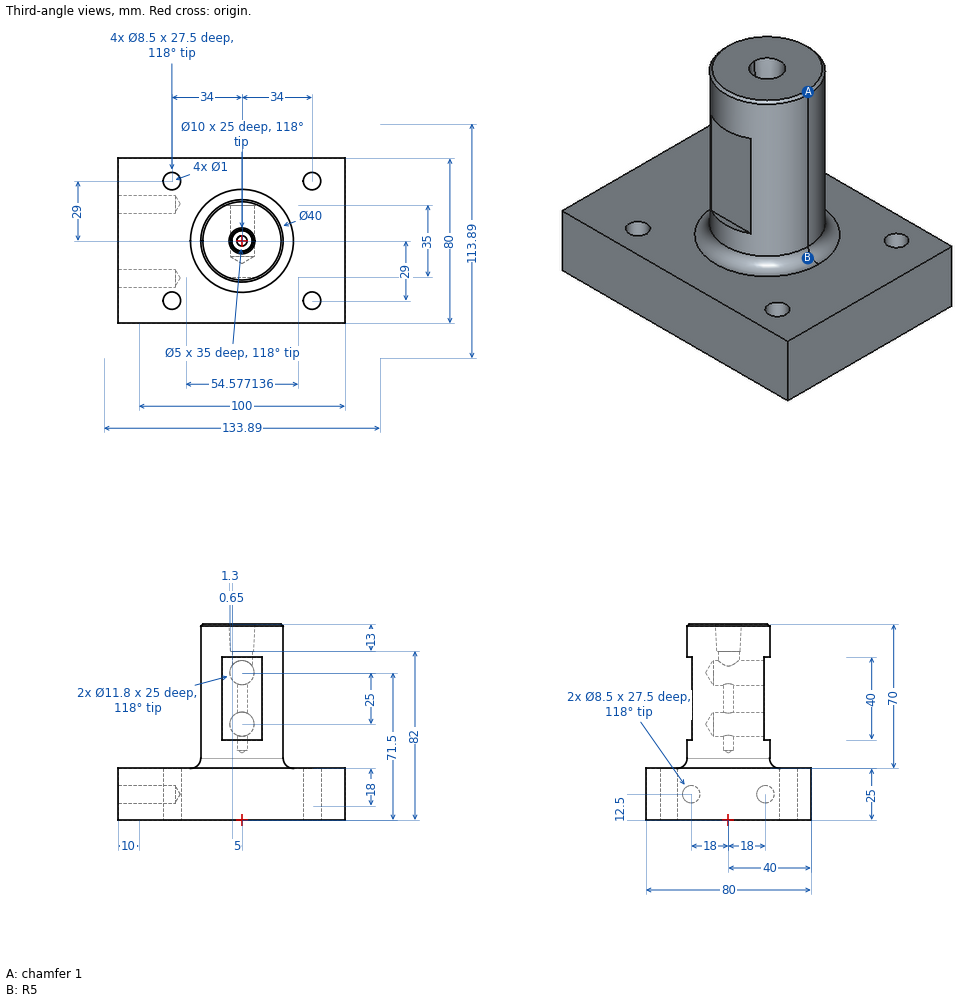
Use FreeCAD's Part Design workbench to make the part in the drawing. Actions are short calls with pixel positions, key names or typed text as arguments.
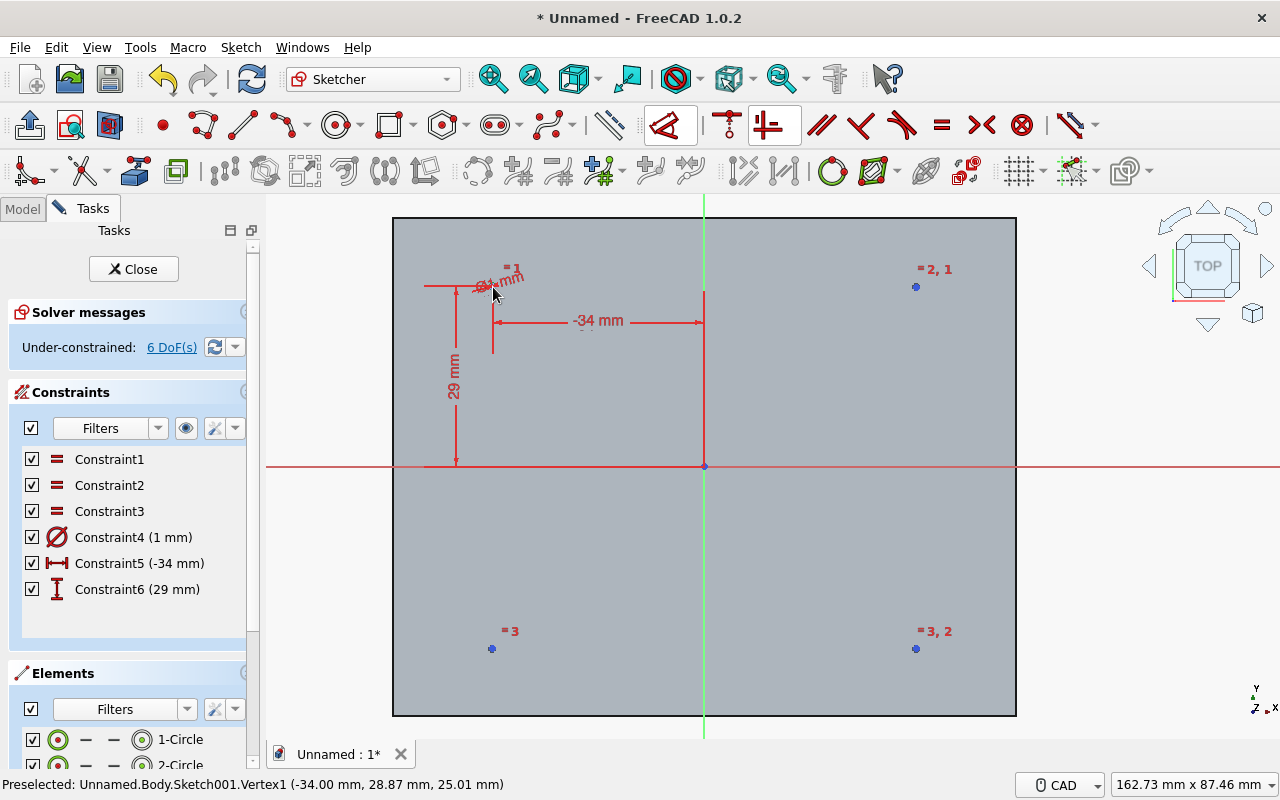
click(916, 287)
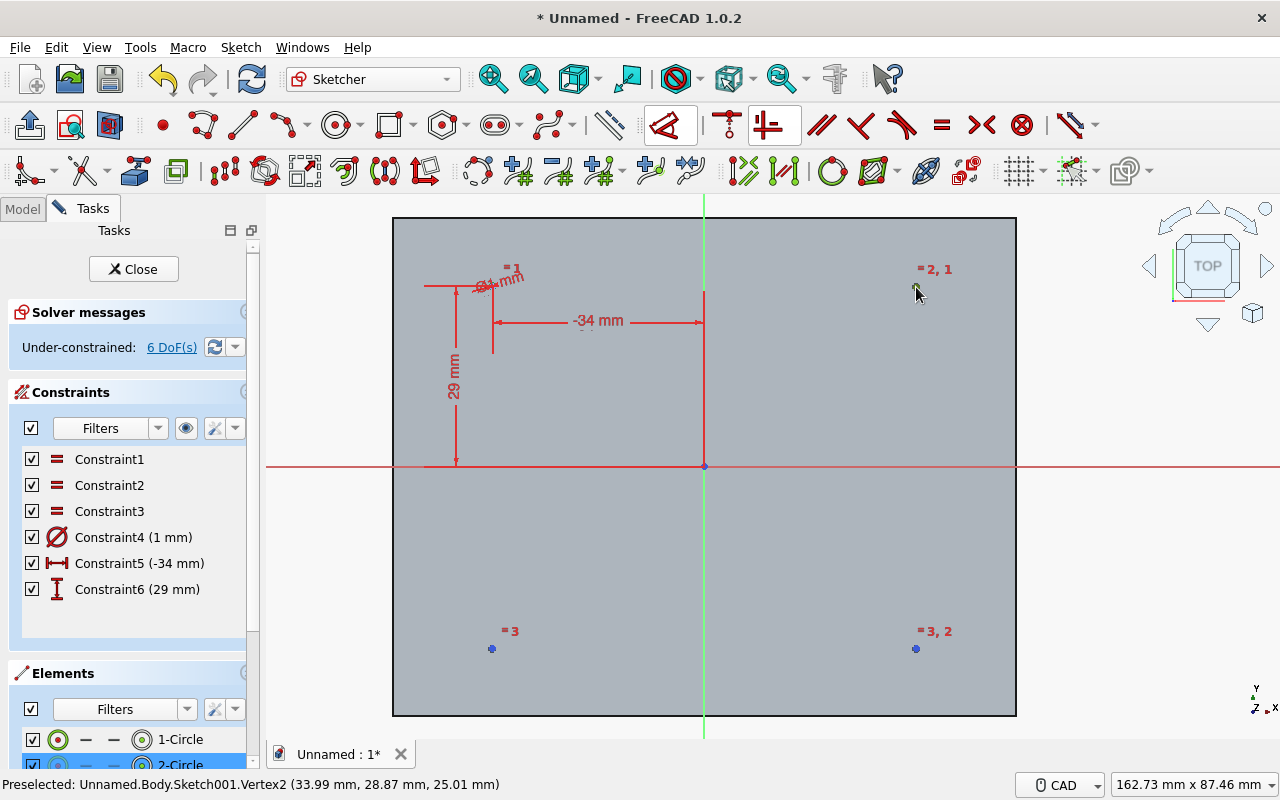
key(l)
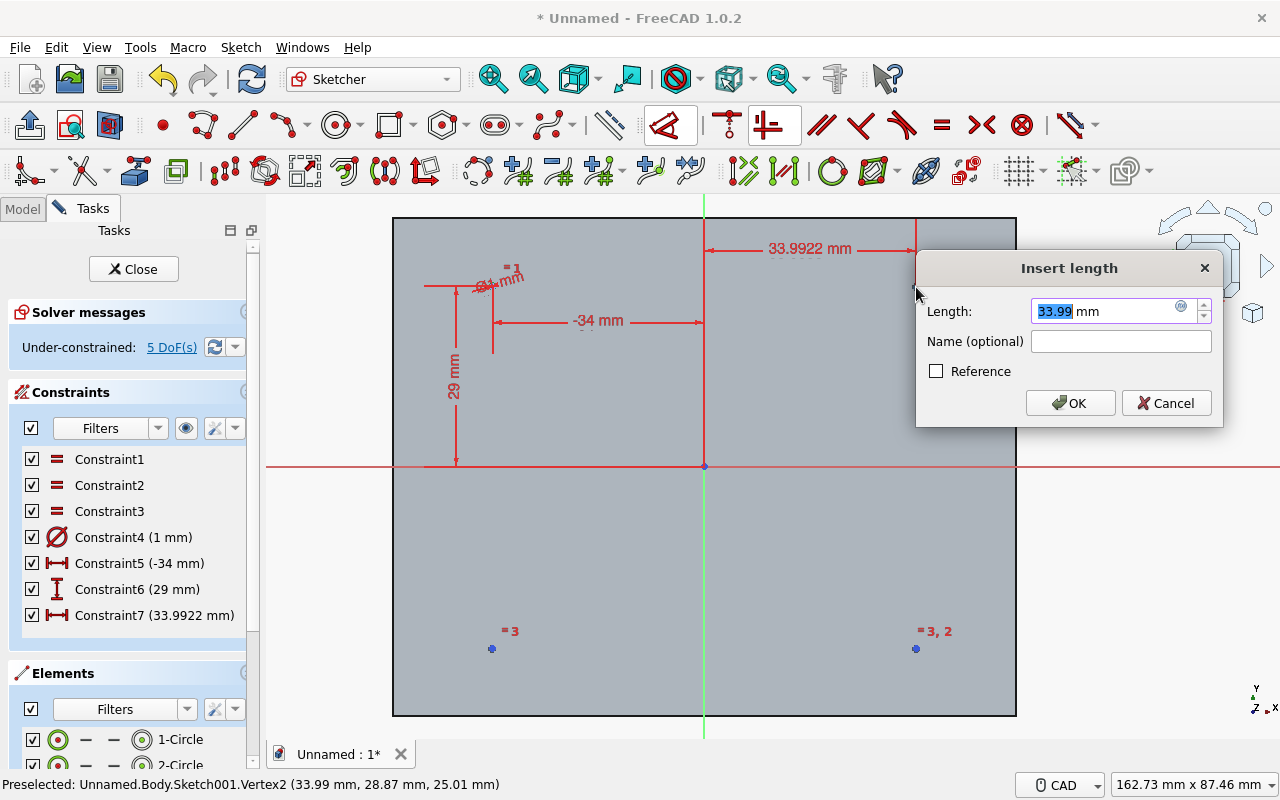
text(34)
key(Return)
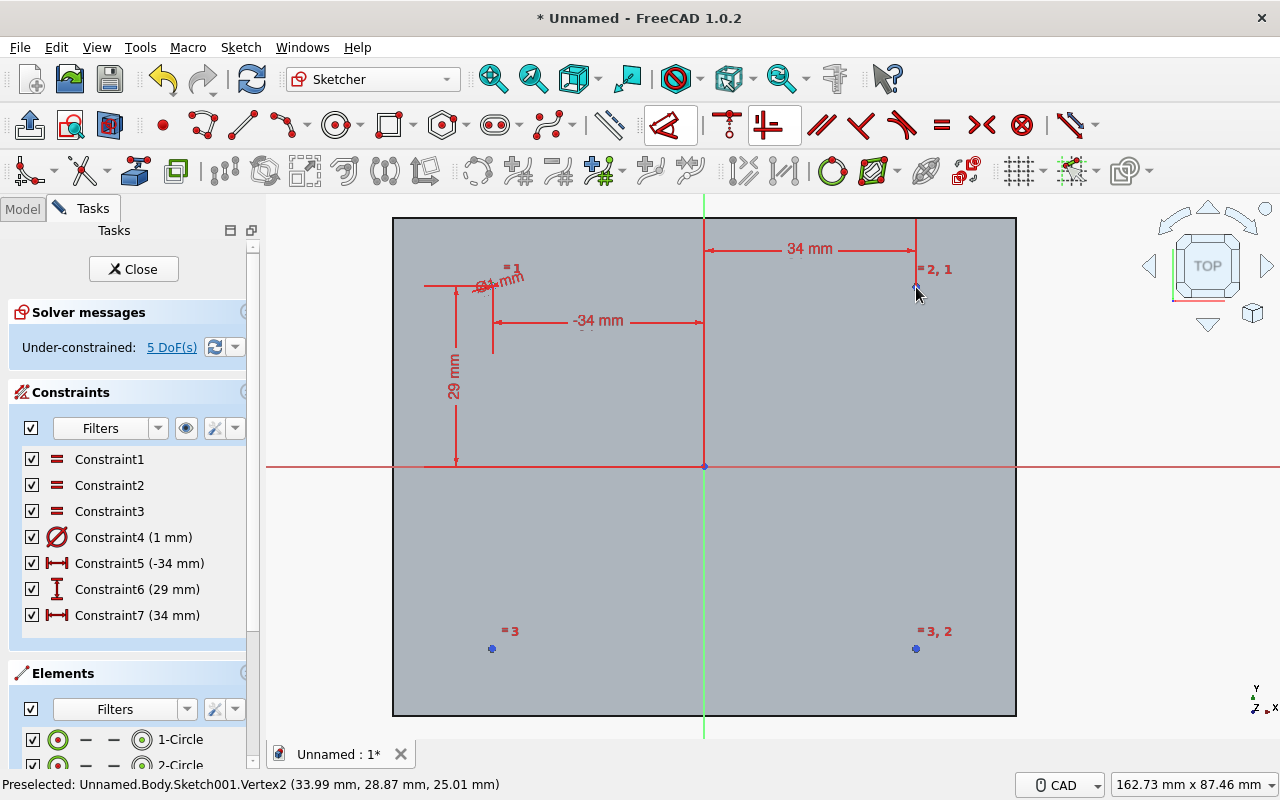
click(916, 287)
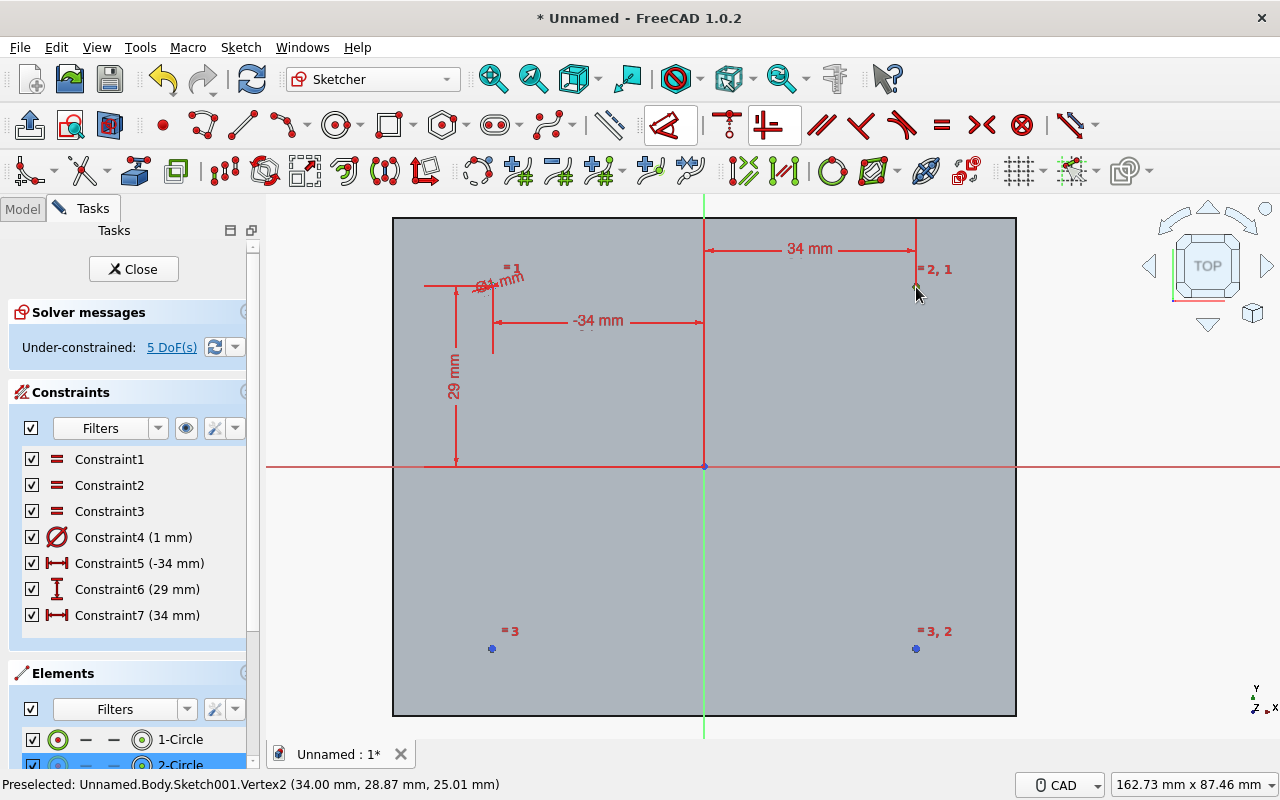
click(692, 126)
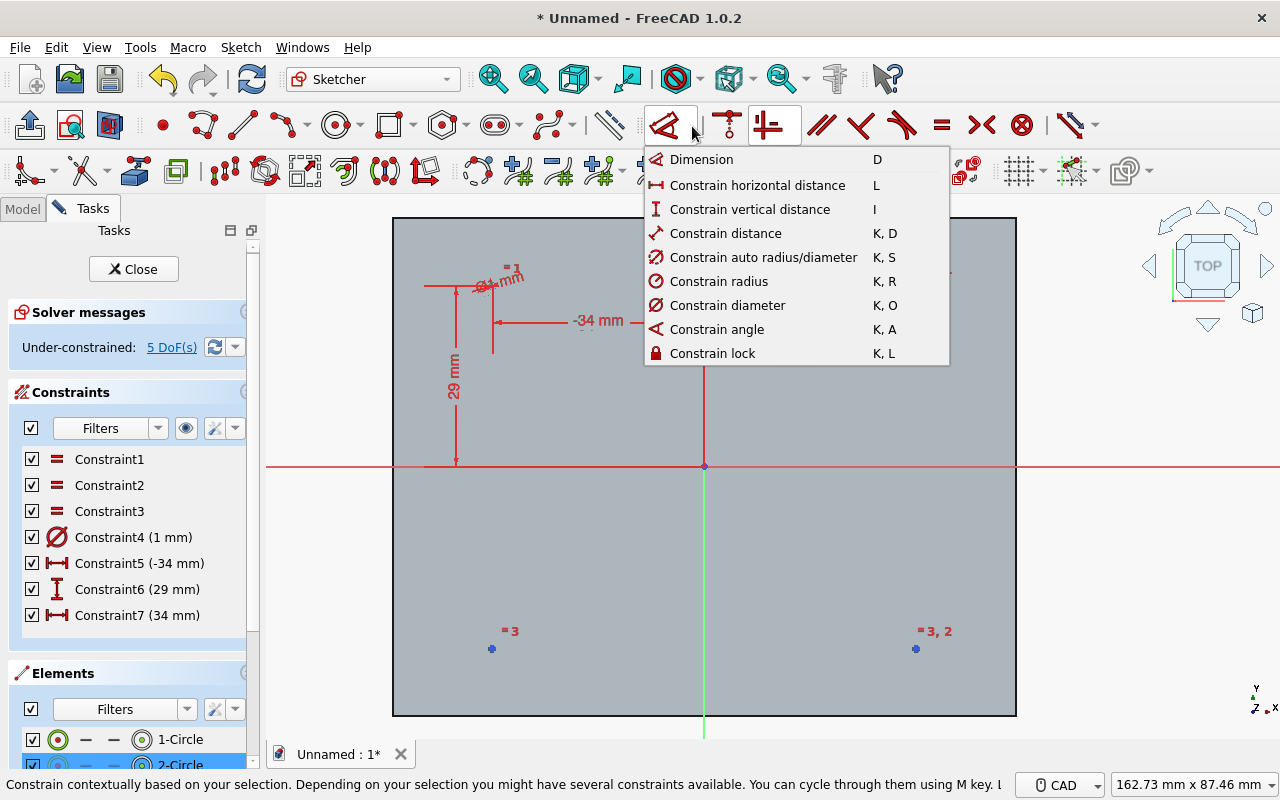
click(797, 209)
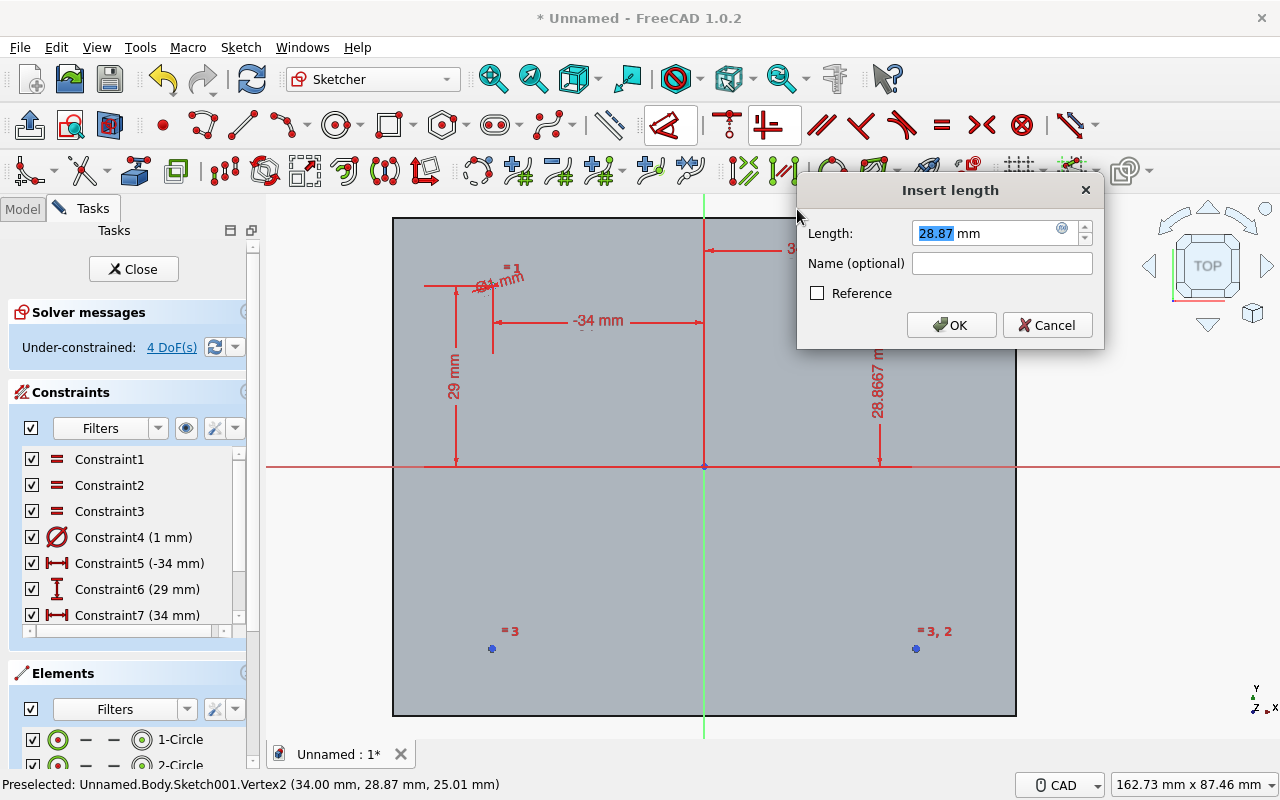
text(29)
key(Return)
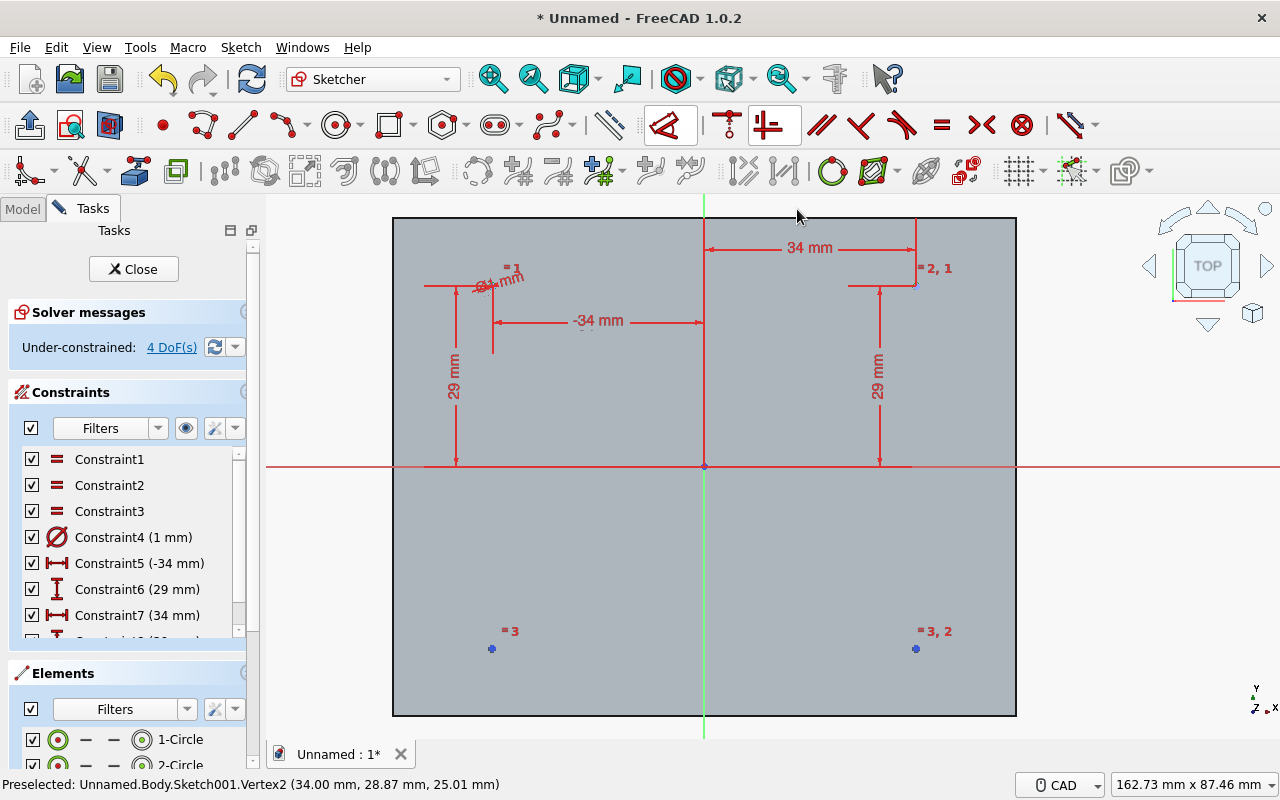
click(916, 649)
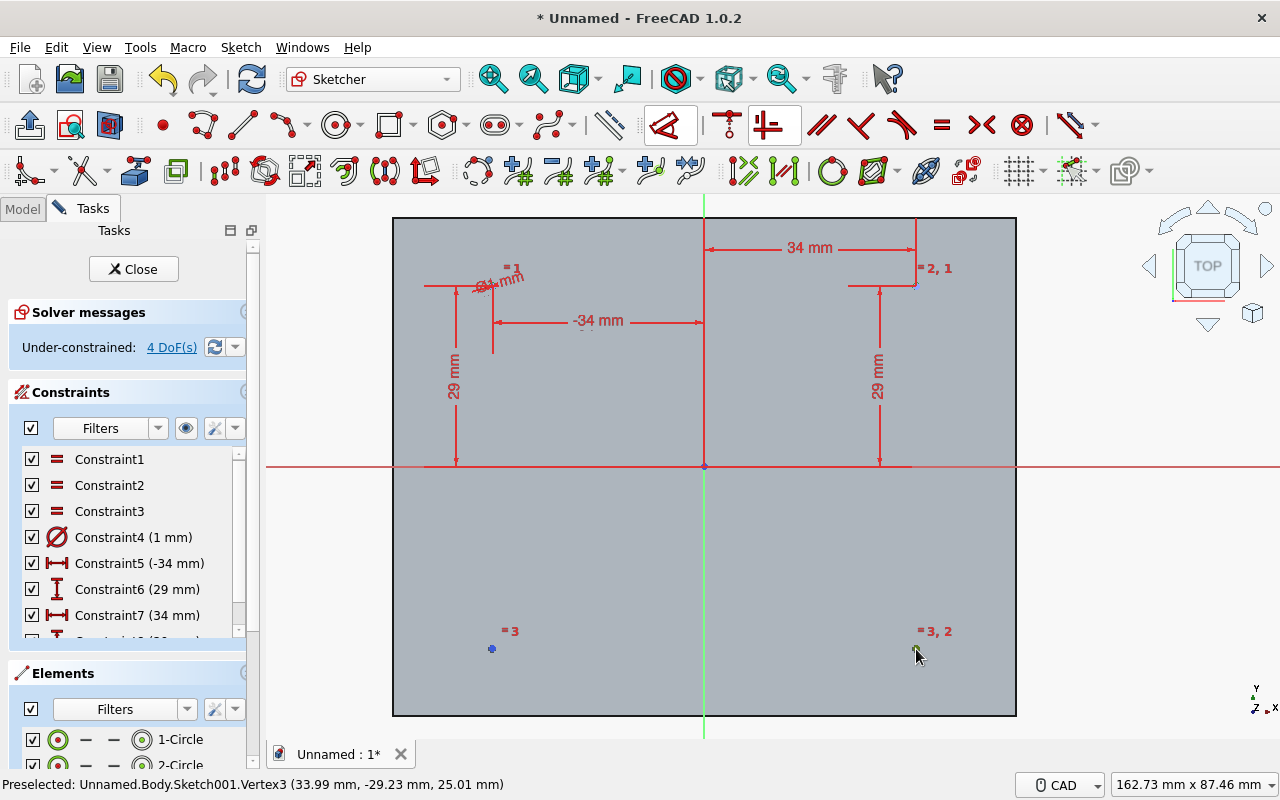
key(l)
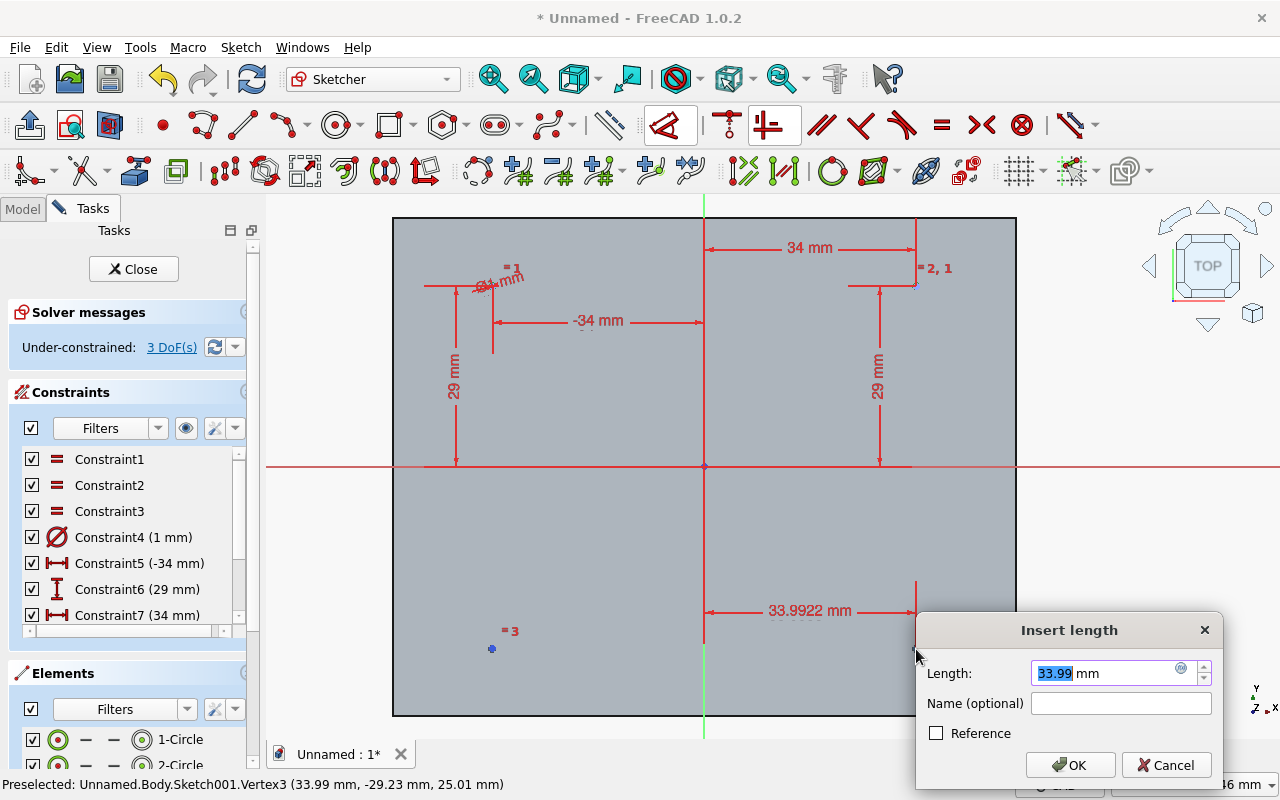
text(34)
key(Return)